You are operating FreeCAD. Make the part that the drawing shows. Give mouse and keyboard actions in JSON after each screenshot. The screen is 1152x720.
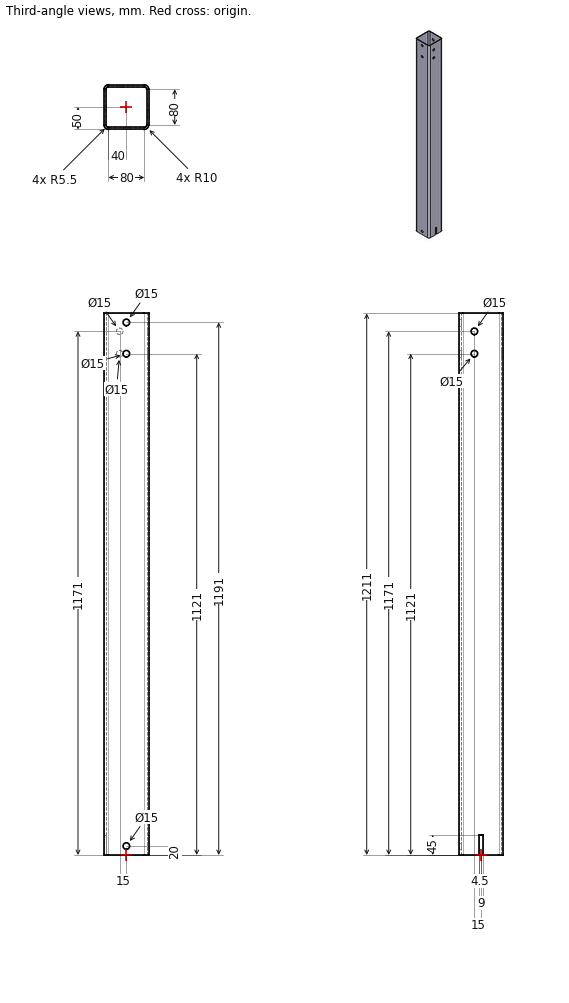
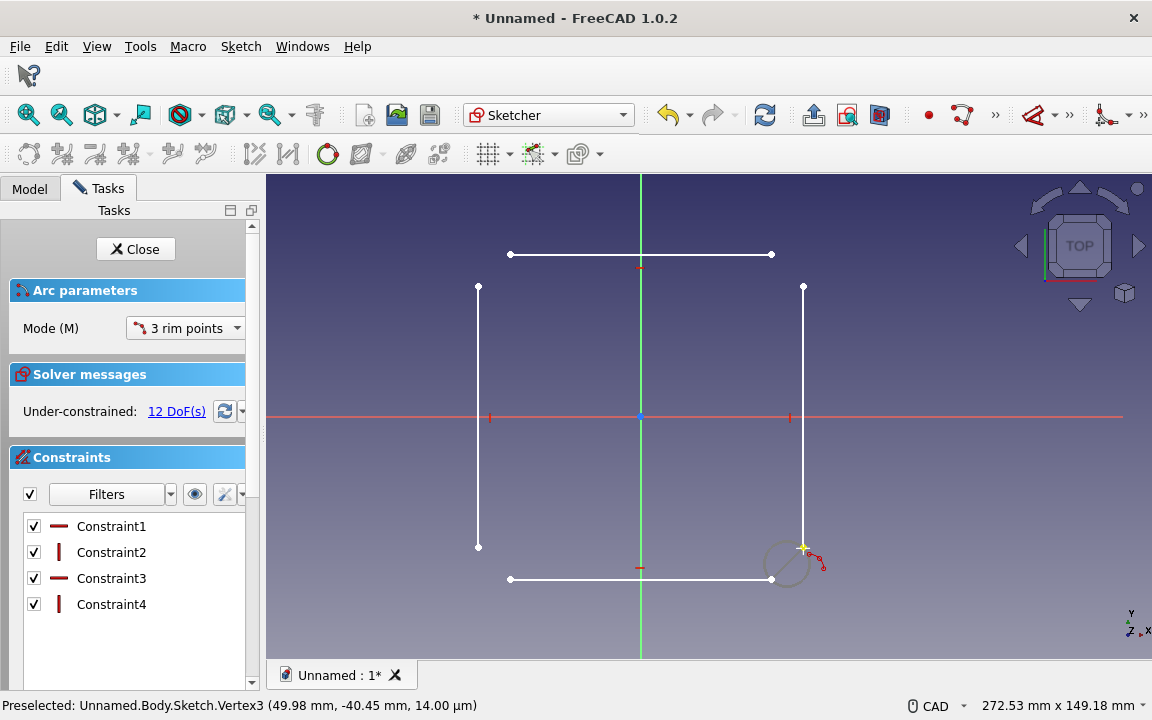
{"action": "scroll", "coordinate": [794, 570], "scroll_direction": "up", "scroll_amount": 3}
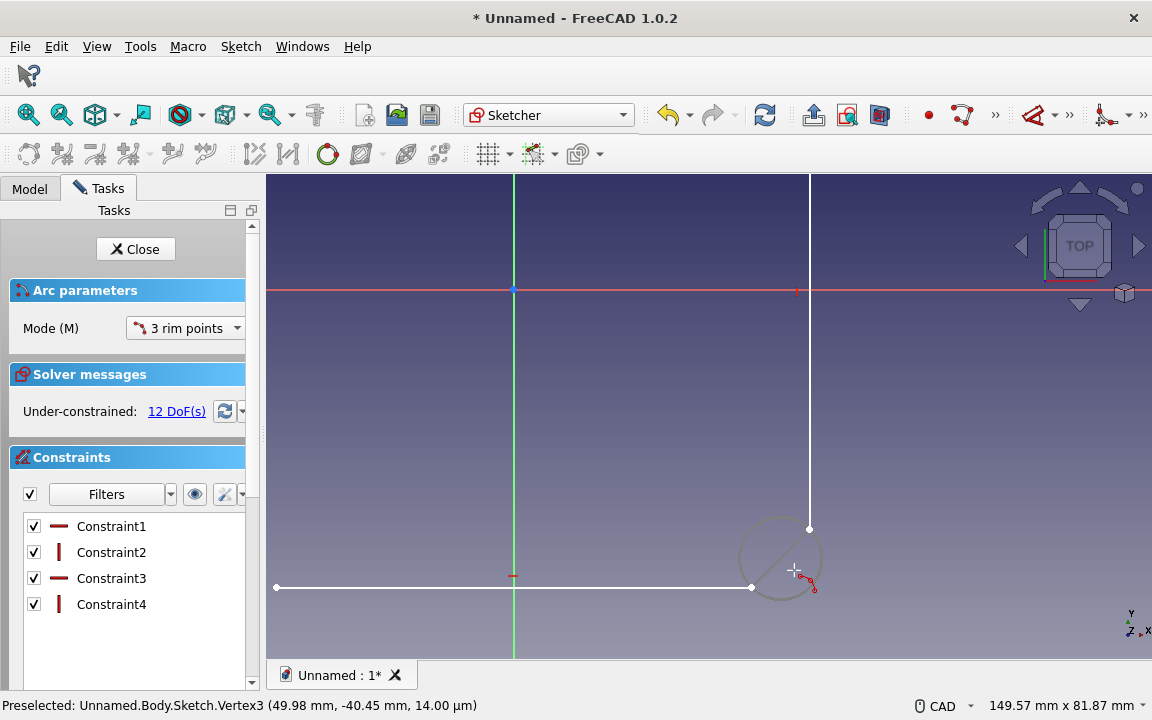
{"action": "left_click", "coordinate": [793, 568]}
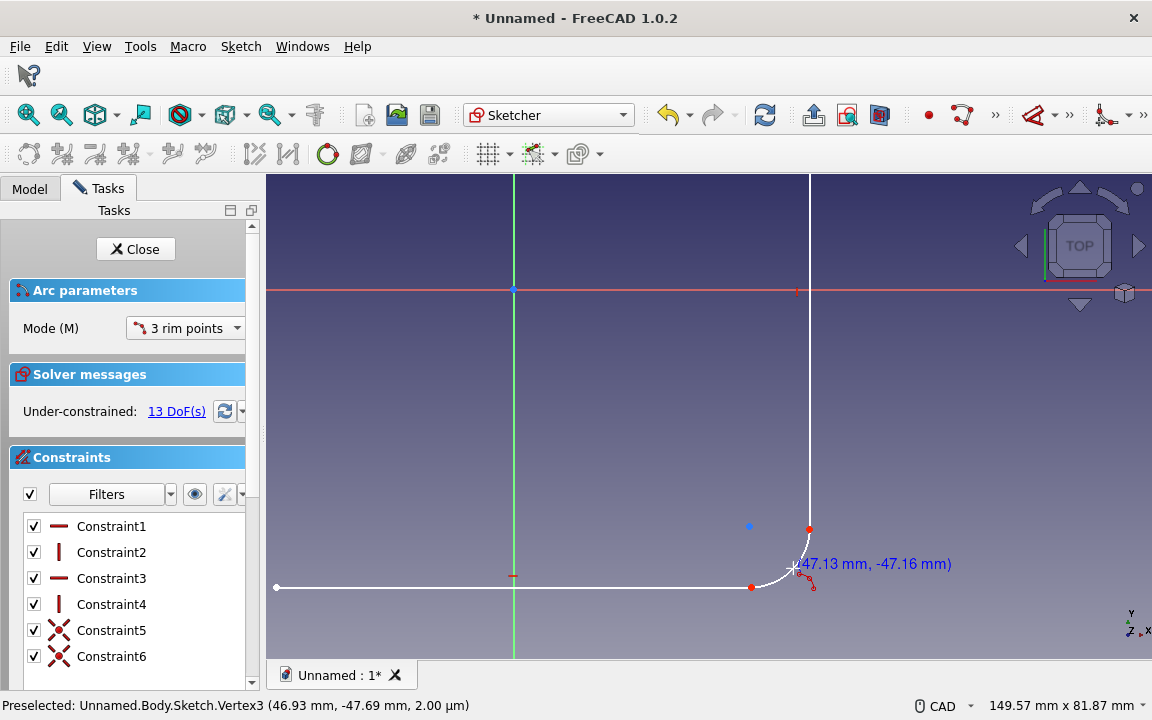
{"action": "scroll", "coordinate": [795, 571], "scroll_direction": "down", "scroll_amount": 3}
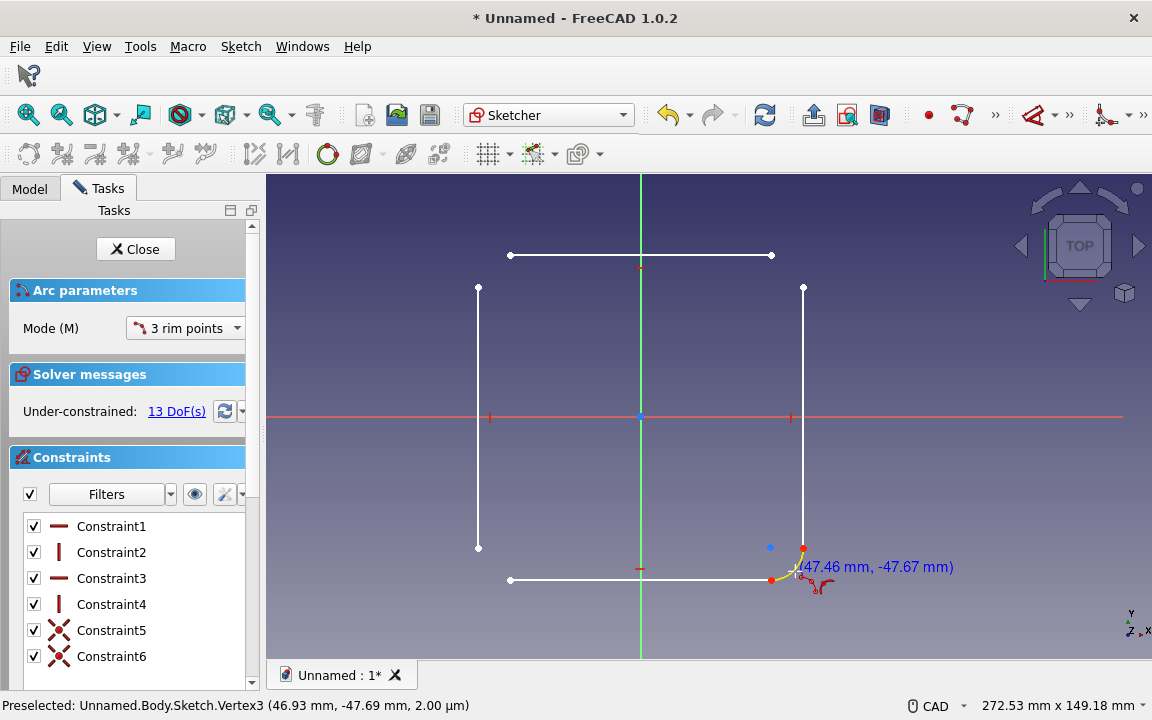
{"action": "left_click", "coordinate": [803, 287]}
{"action": "left_click", "coordinate": [771, 255]}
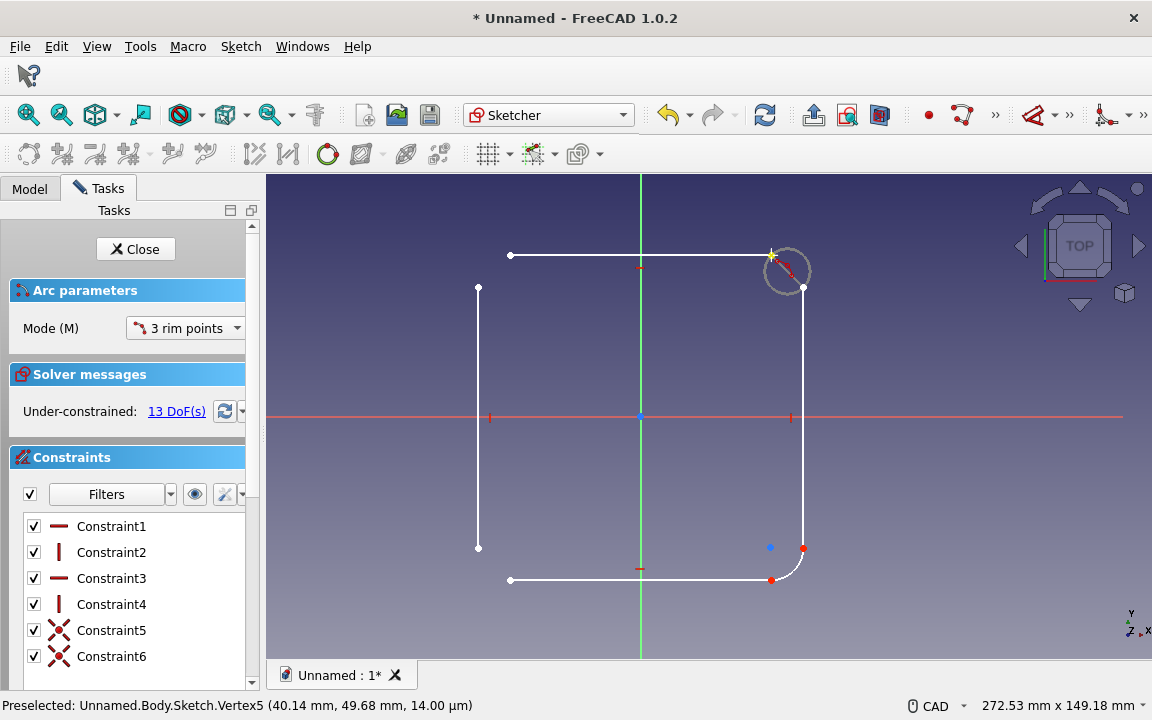
{"action": "scroll", "coordinate": [794, 264], "scroll_direction": "up", "scroll_amount": 3}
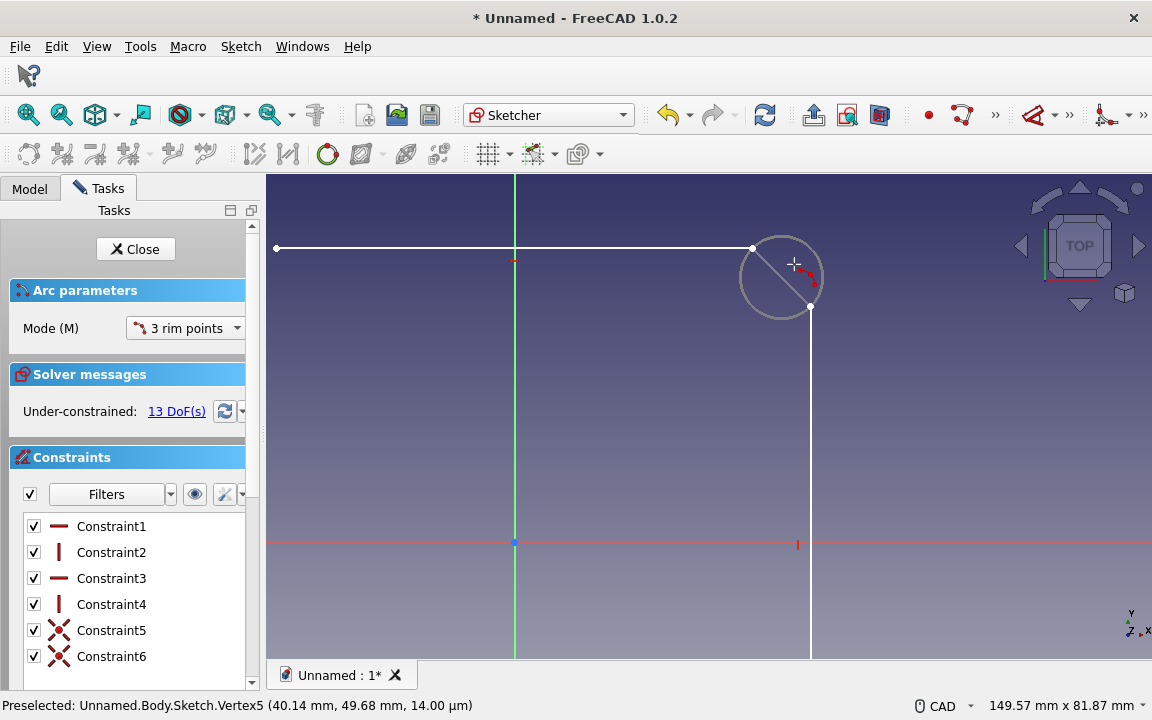
{"action": "left_click", "coordinate": [794, 264]}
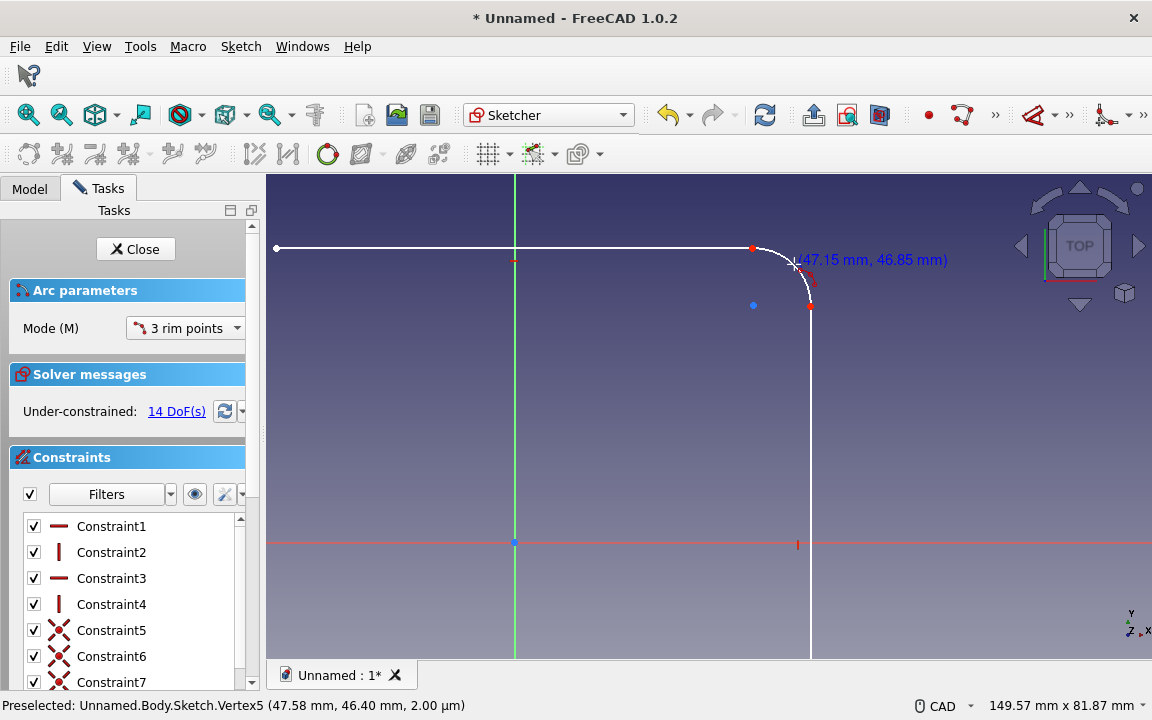
{"action": "scroll", "coordinate": [794, 263], "scroll_direction": "down", "scroll_amount": 3}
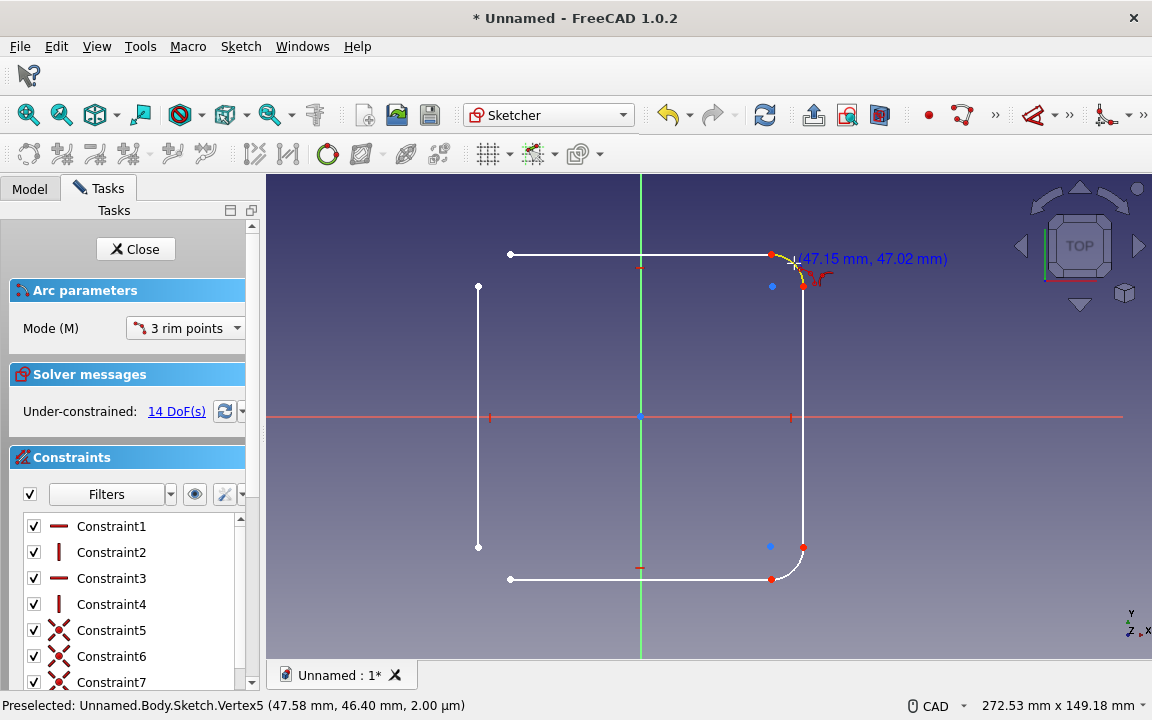
{"action": "left_click", "coordinate": [510, 255]}
{"action": "left_click", "coordinate": [478, 287]}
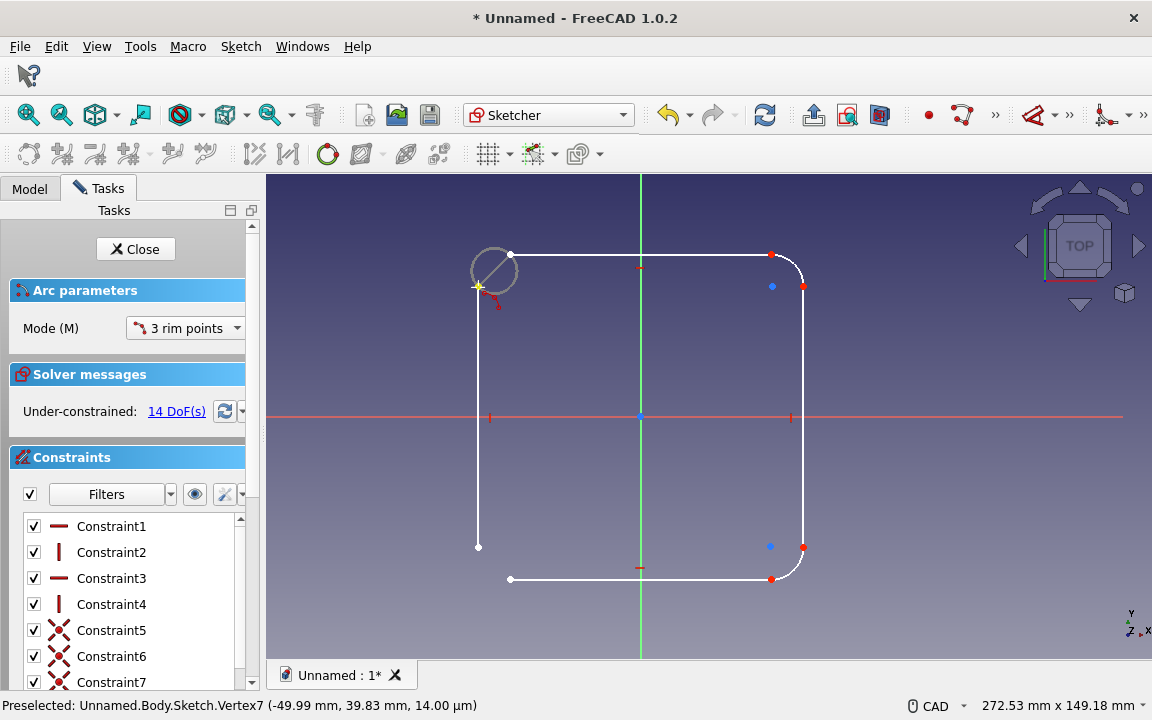
{"action": "scroll", "coordinate": [488, 263], "scroll_direction": "up", "scroll_amount": 3}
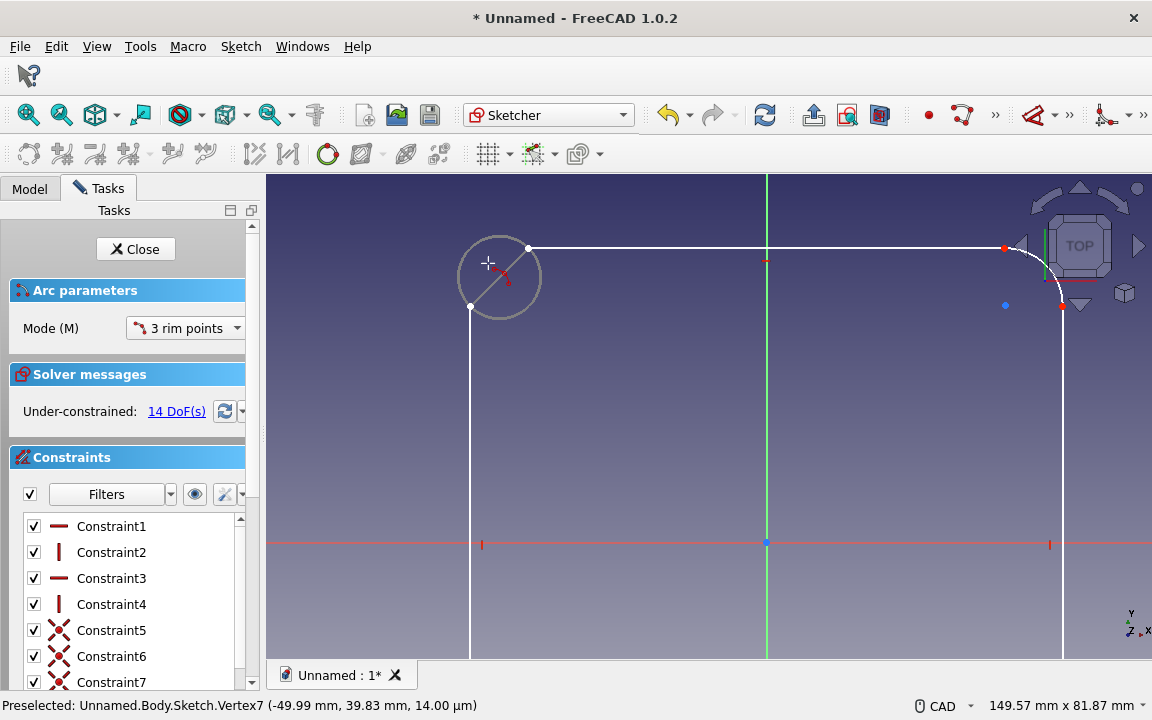
{"action": "left_click", "coordinate": [488, 264]}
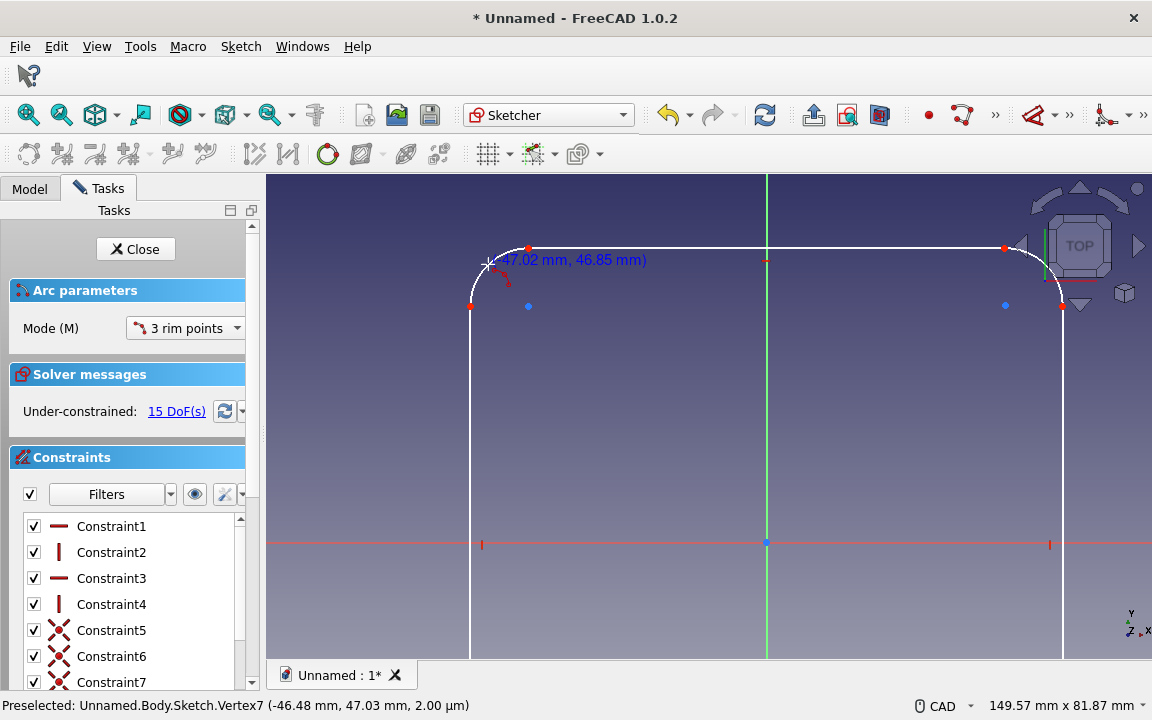
{"action": "scroll", "coordinate": [487, 263], "scroll_direction": "down", "scroll_amount": 3}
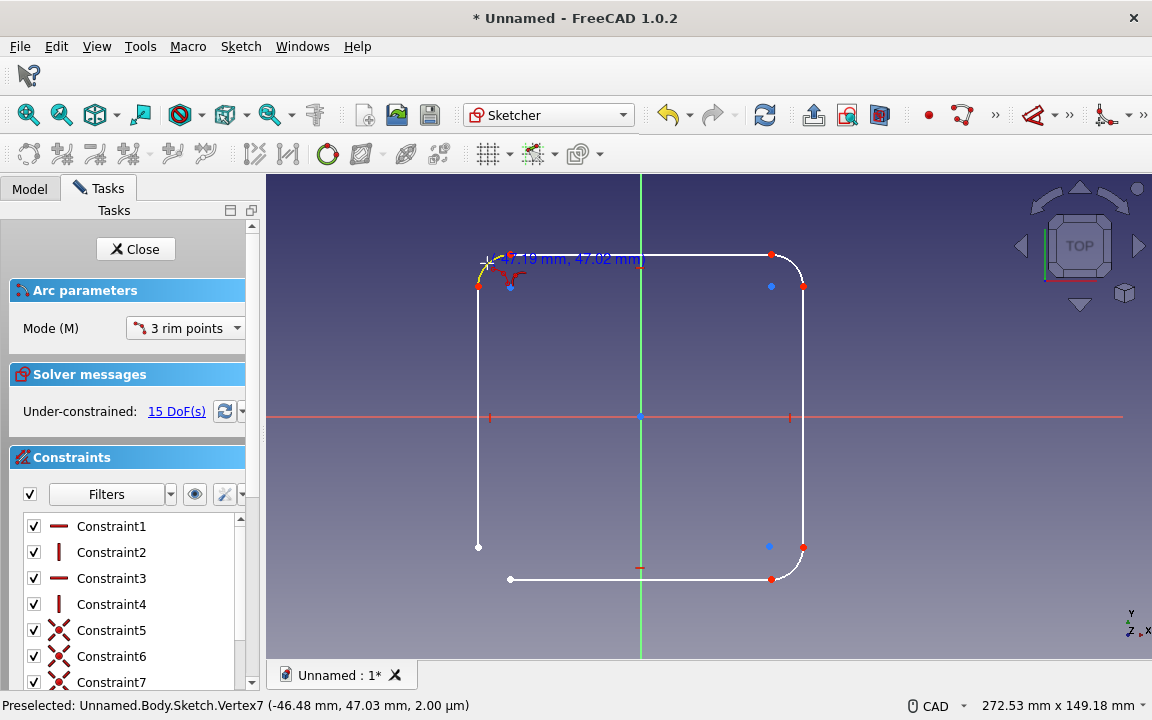
{"action": "left_click", "coordinate": [478, 548]}
{"action": "left_click", "coordinate": [510, 580]}